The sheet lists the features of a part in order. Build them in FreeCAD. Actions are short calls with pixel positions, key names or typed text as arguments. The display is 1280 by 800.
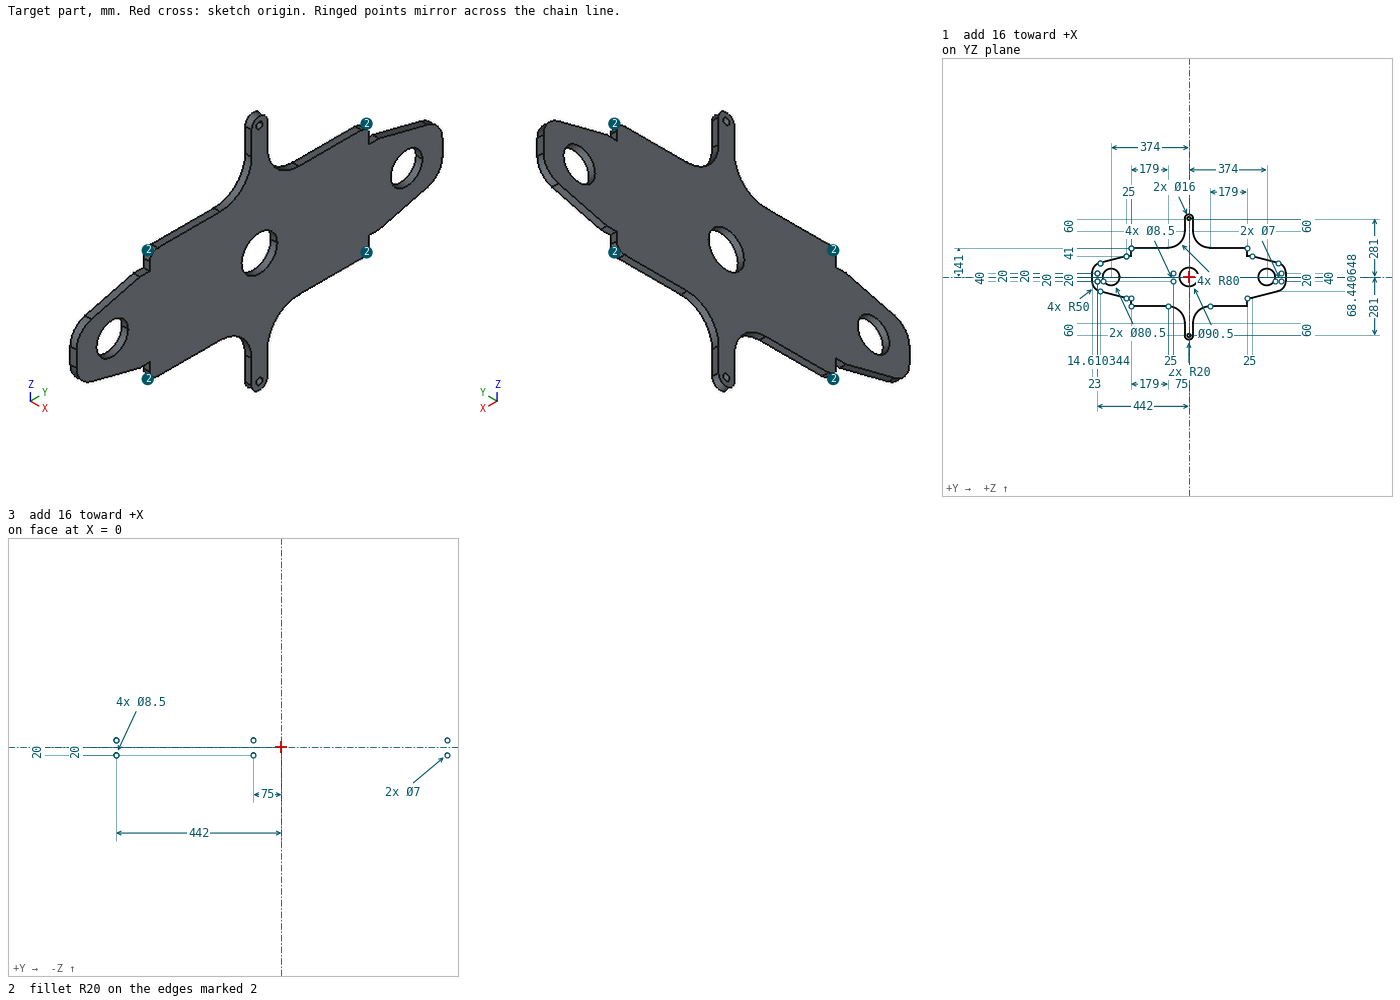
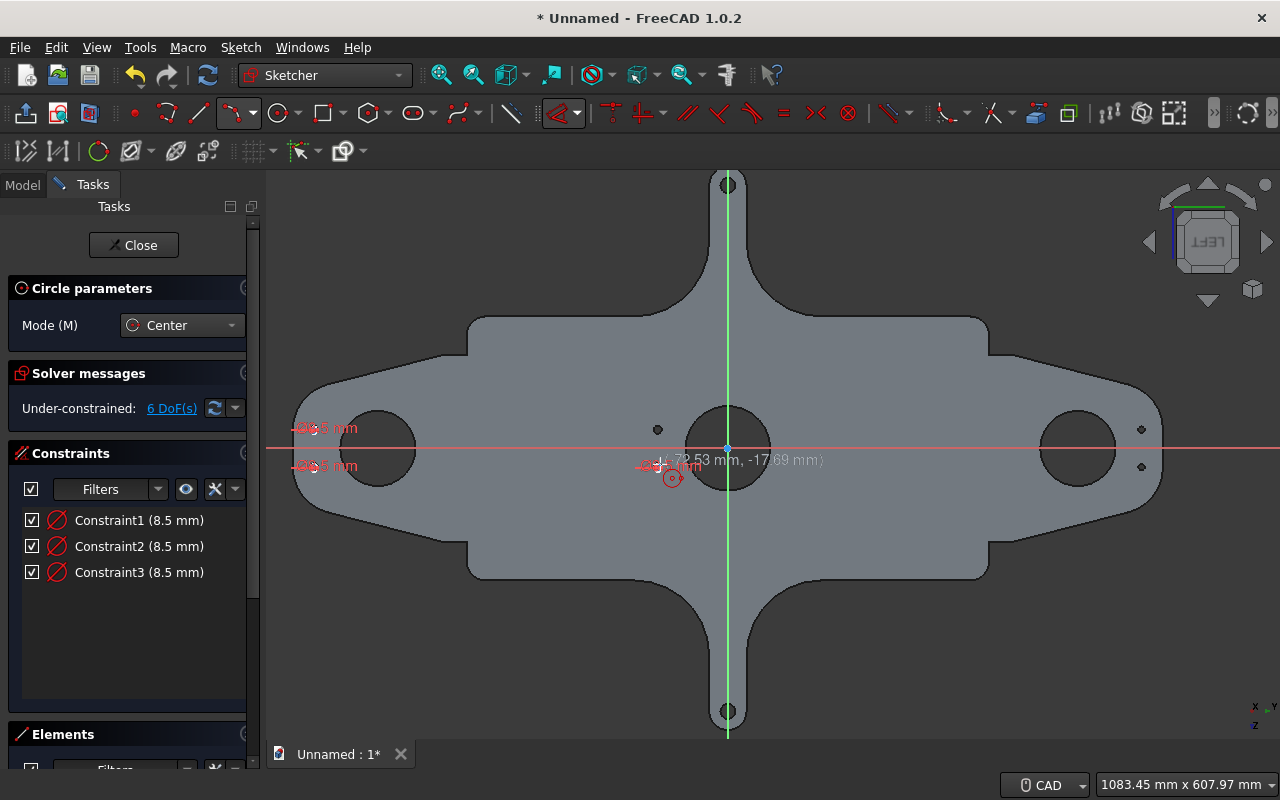
scroll(658, 430, up, 9)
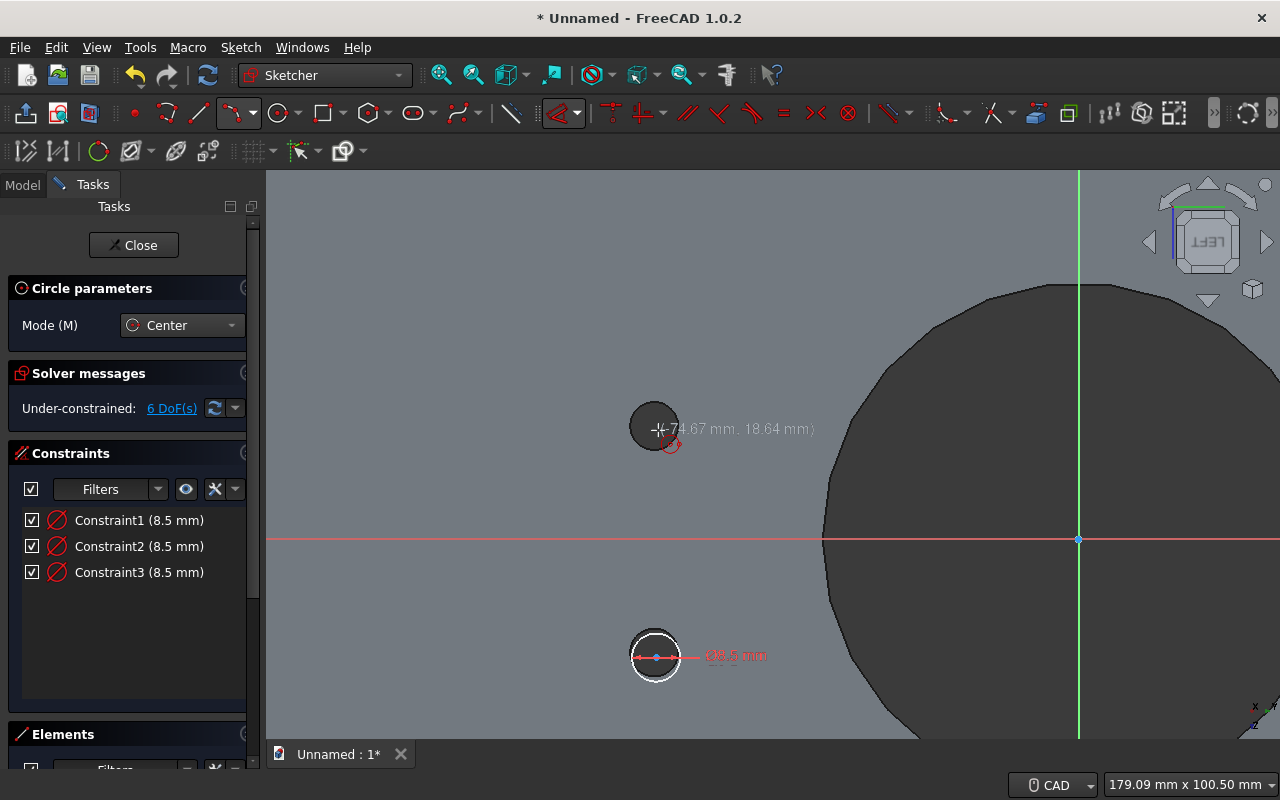
scroll(658, 444, down, 11)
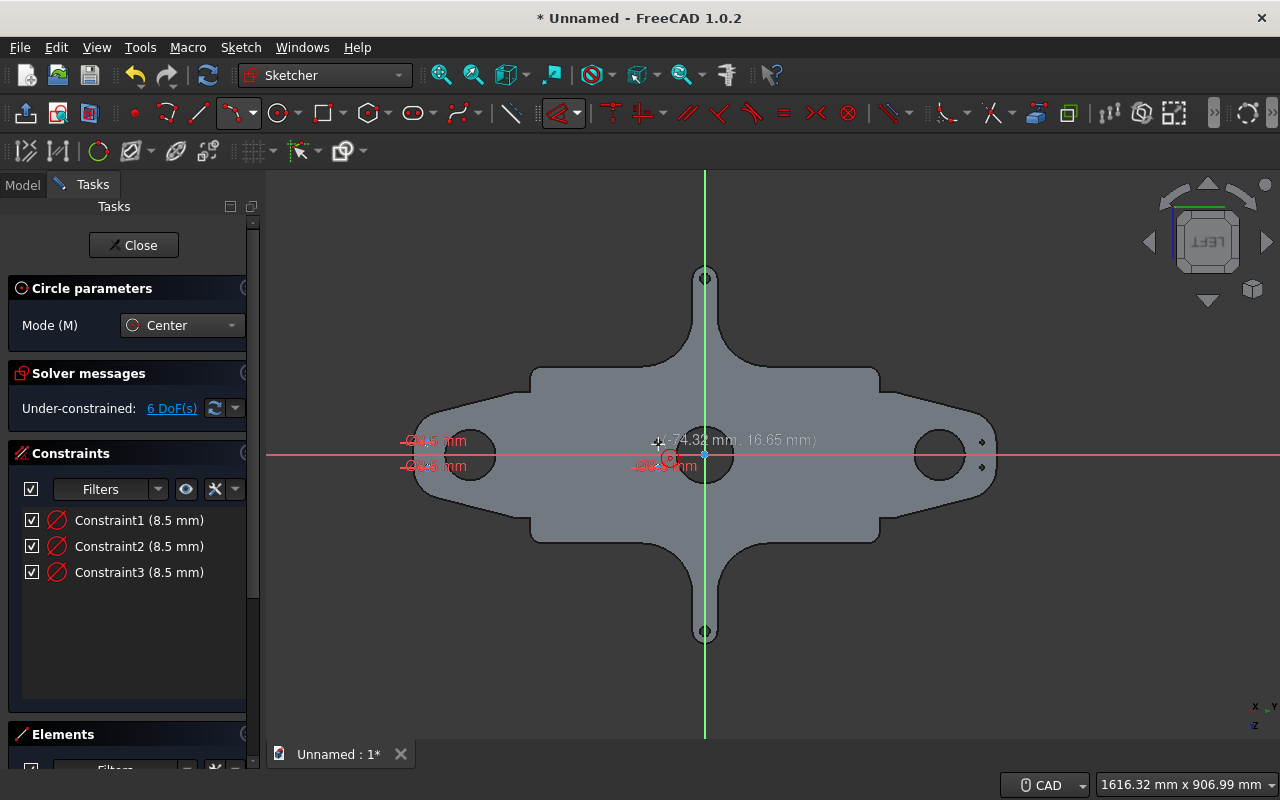
scroll(658, 442, up, 2)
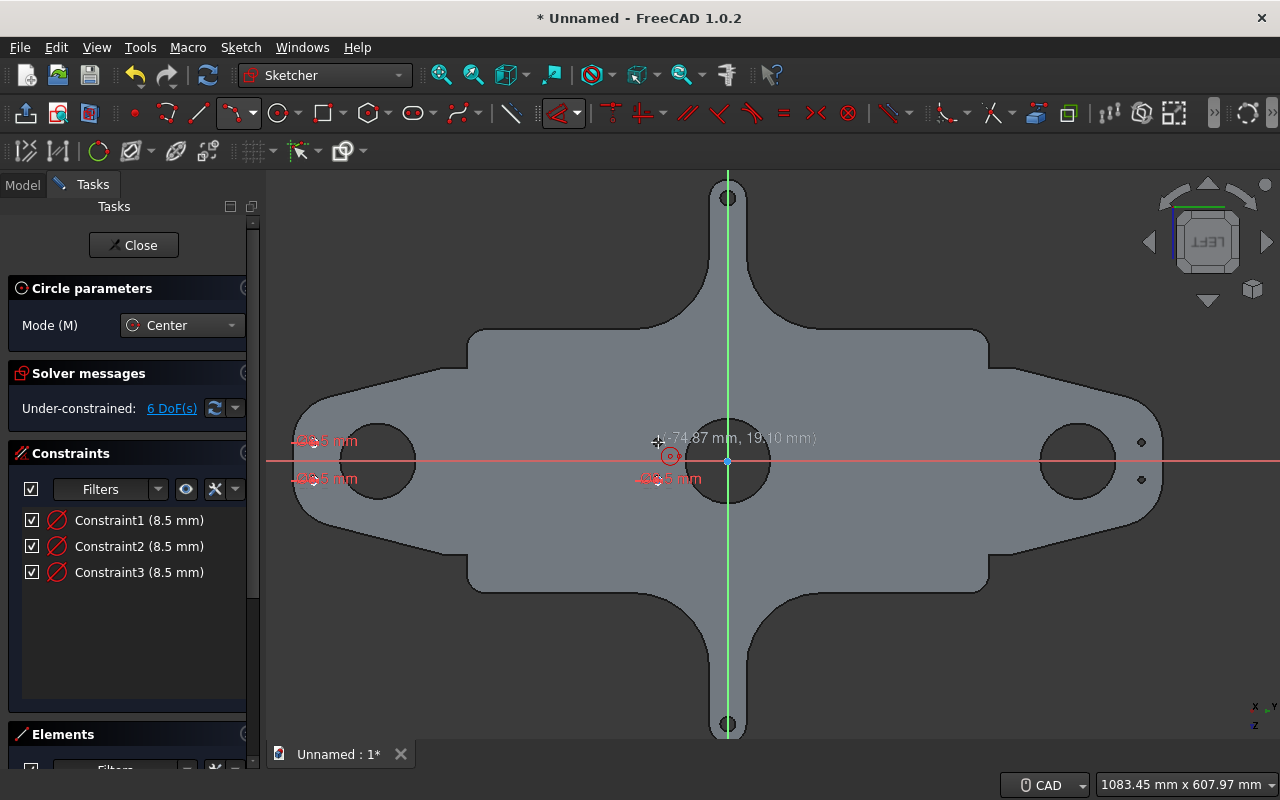
click(658, 442)
move(661, 440)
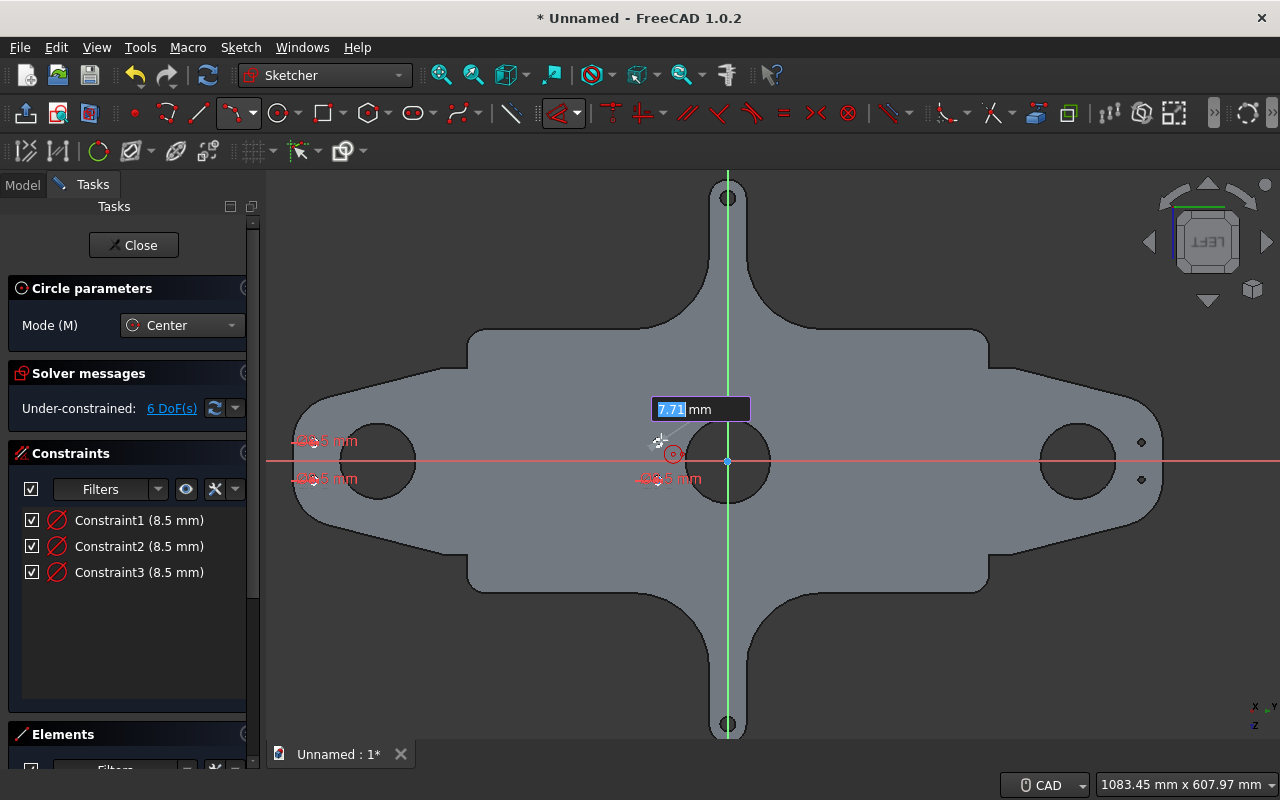
text(8.5)
key(Return)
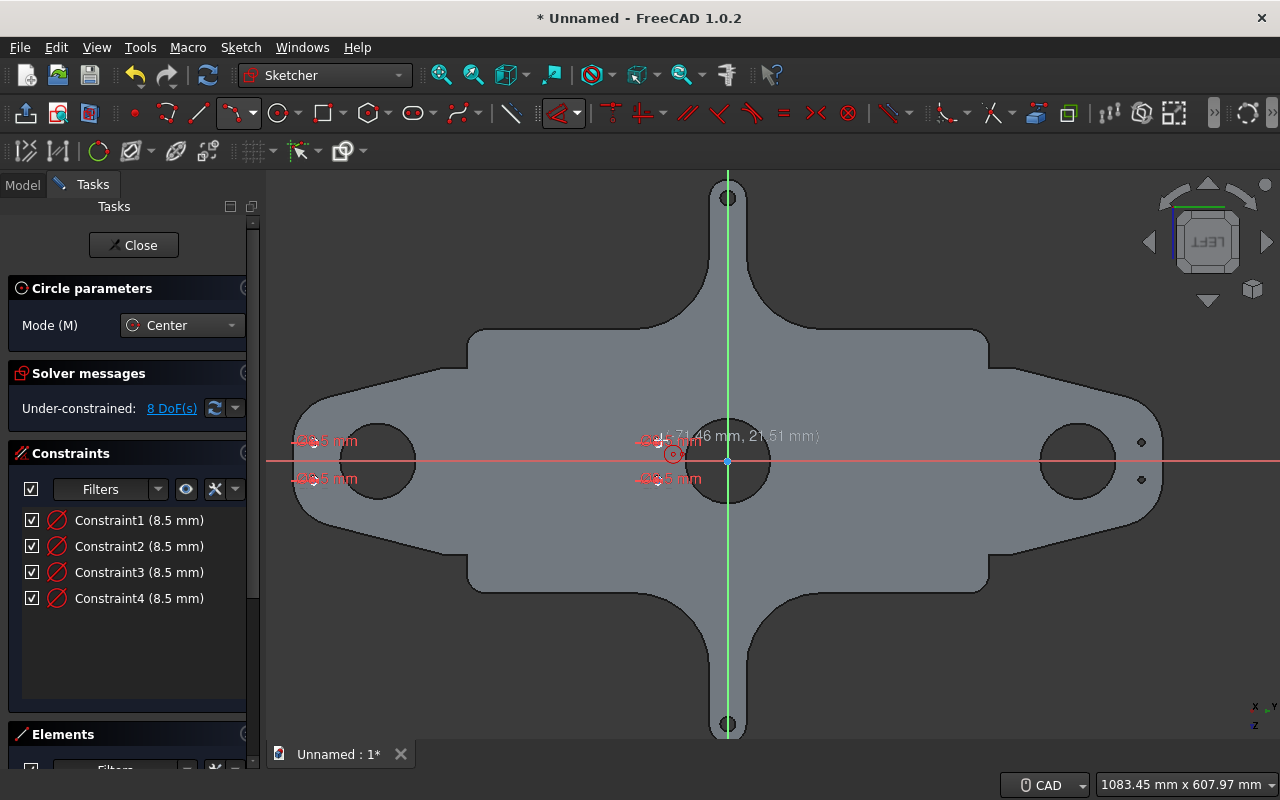
scroll(658, 441, down, 2)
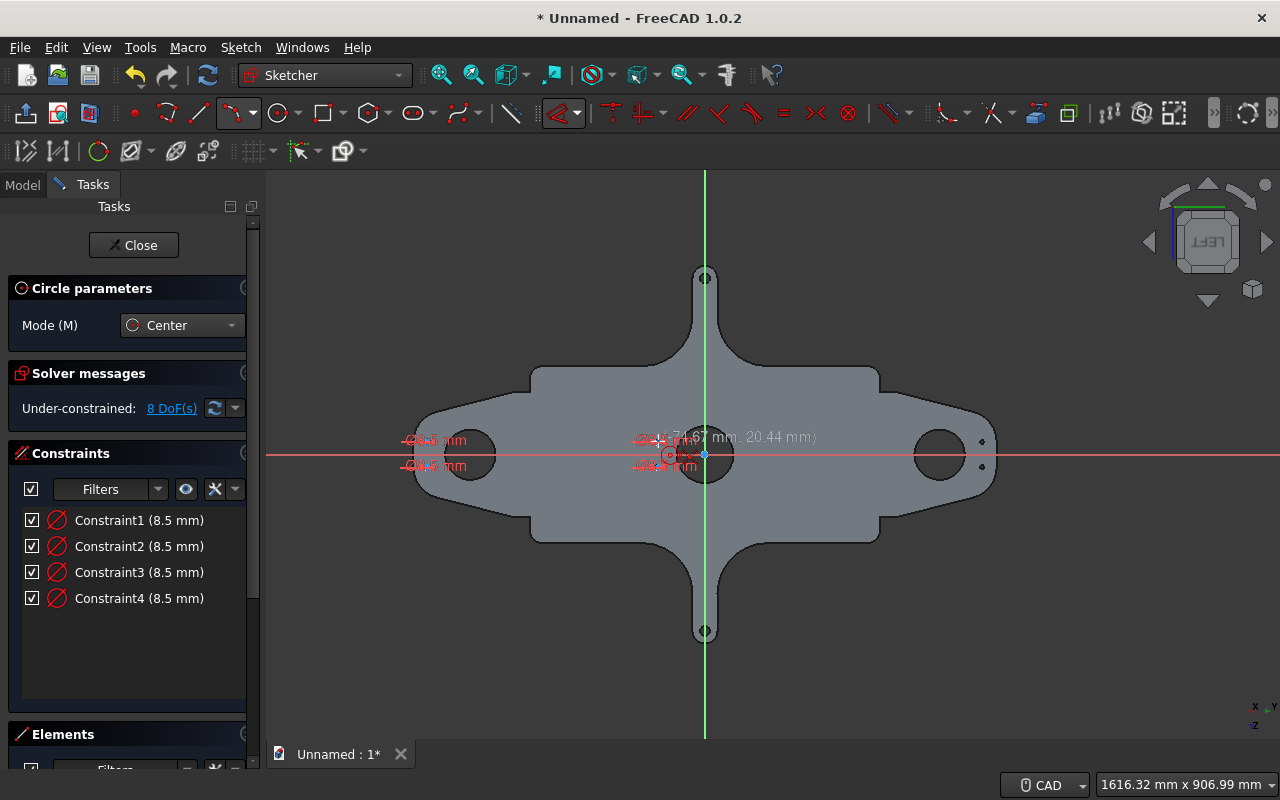
scroll(982, 467, up, 12)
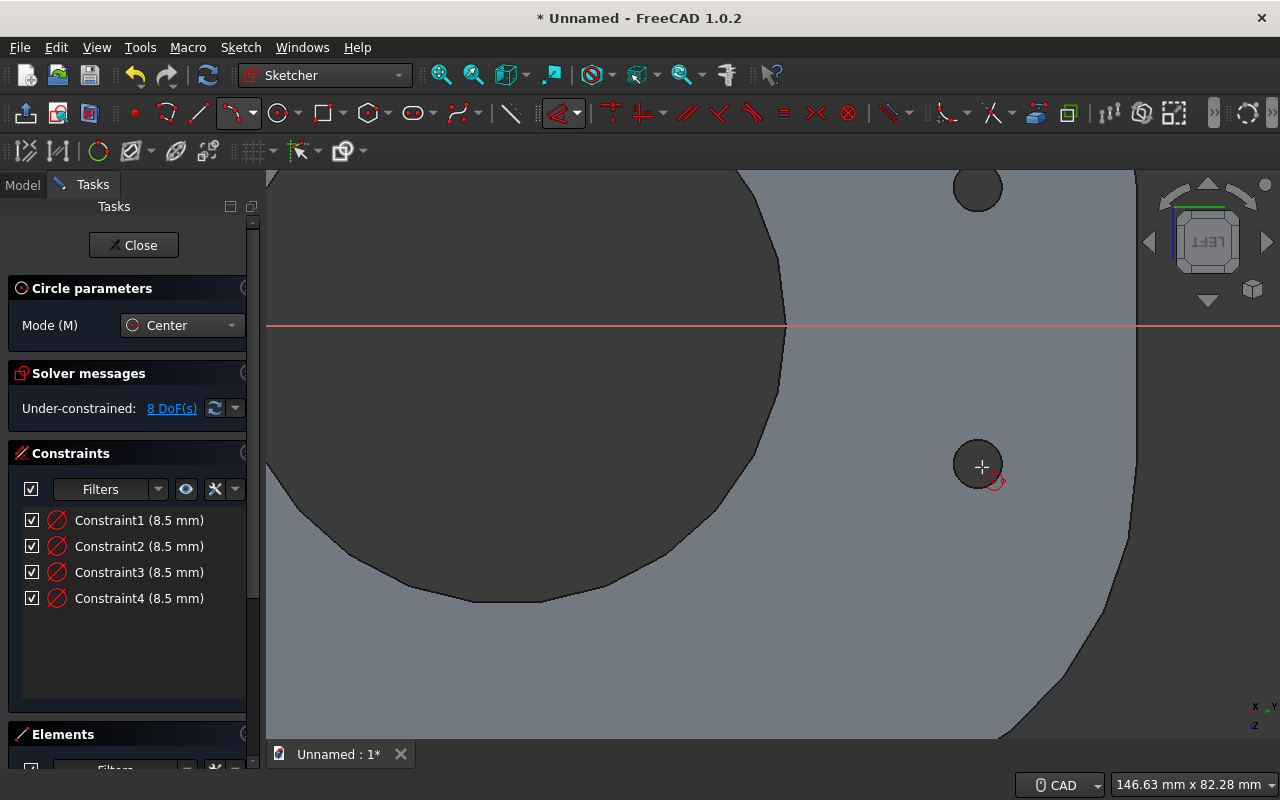
scroll(982, 467, down, 12)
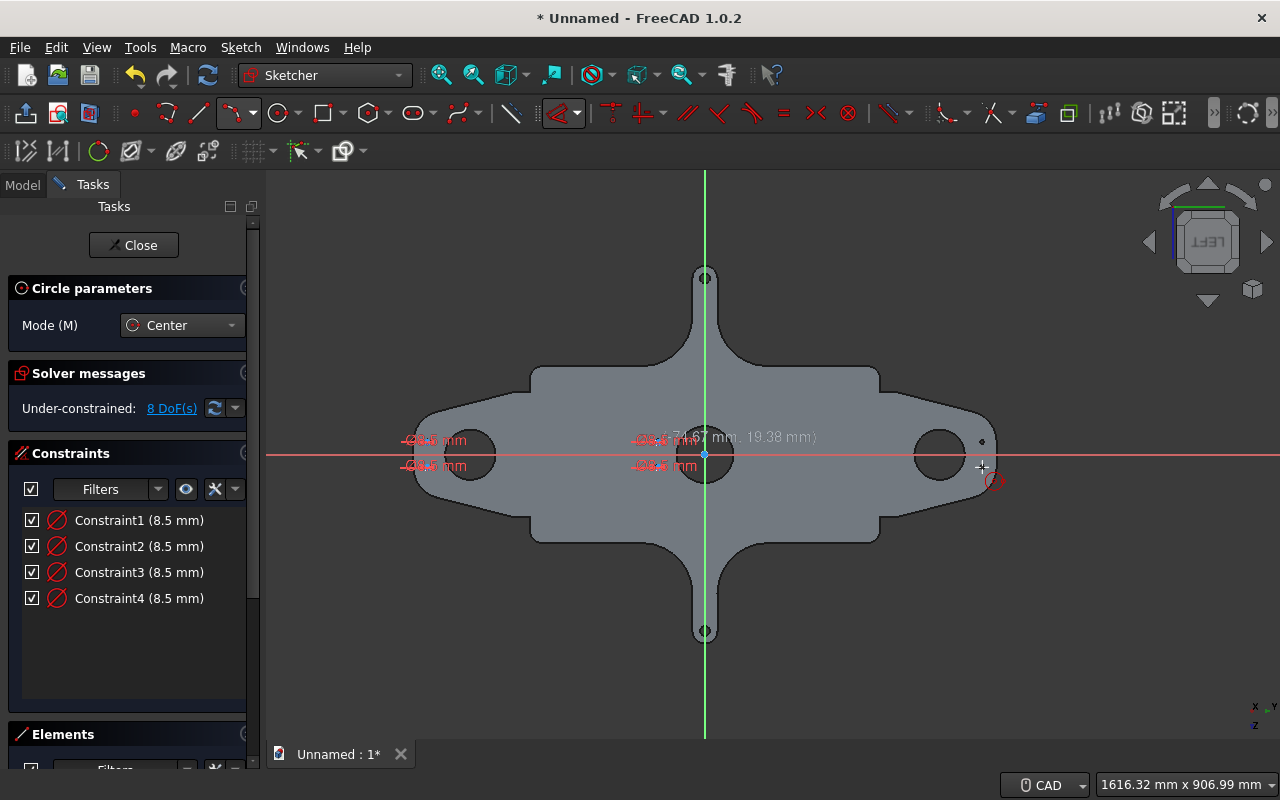
scroll(982, 467, up, 2)